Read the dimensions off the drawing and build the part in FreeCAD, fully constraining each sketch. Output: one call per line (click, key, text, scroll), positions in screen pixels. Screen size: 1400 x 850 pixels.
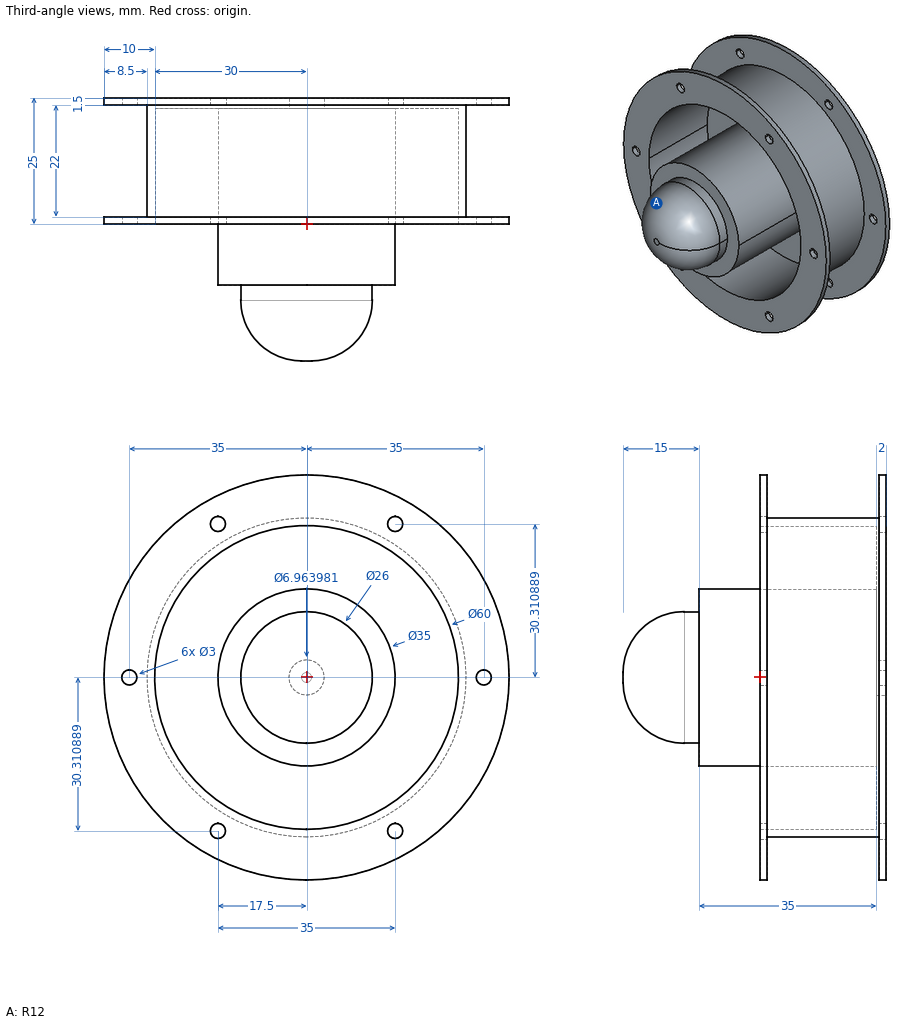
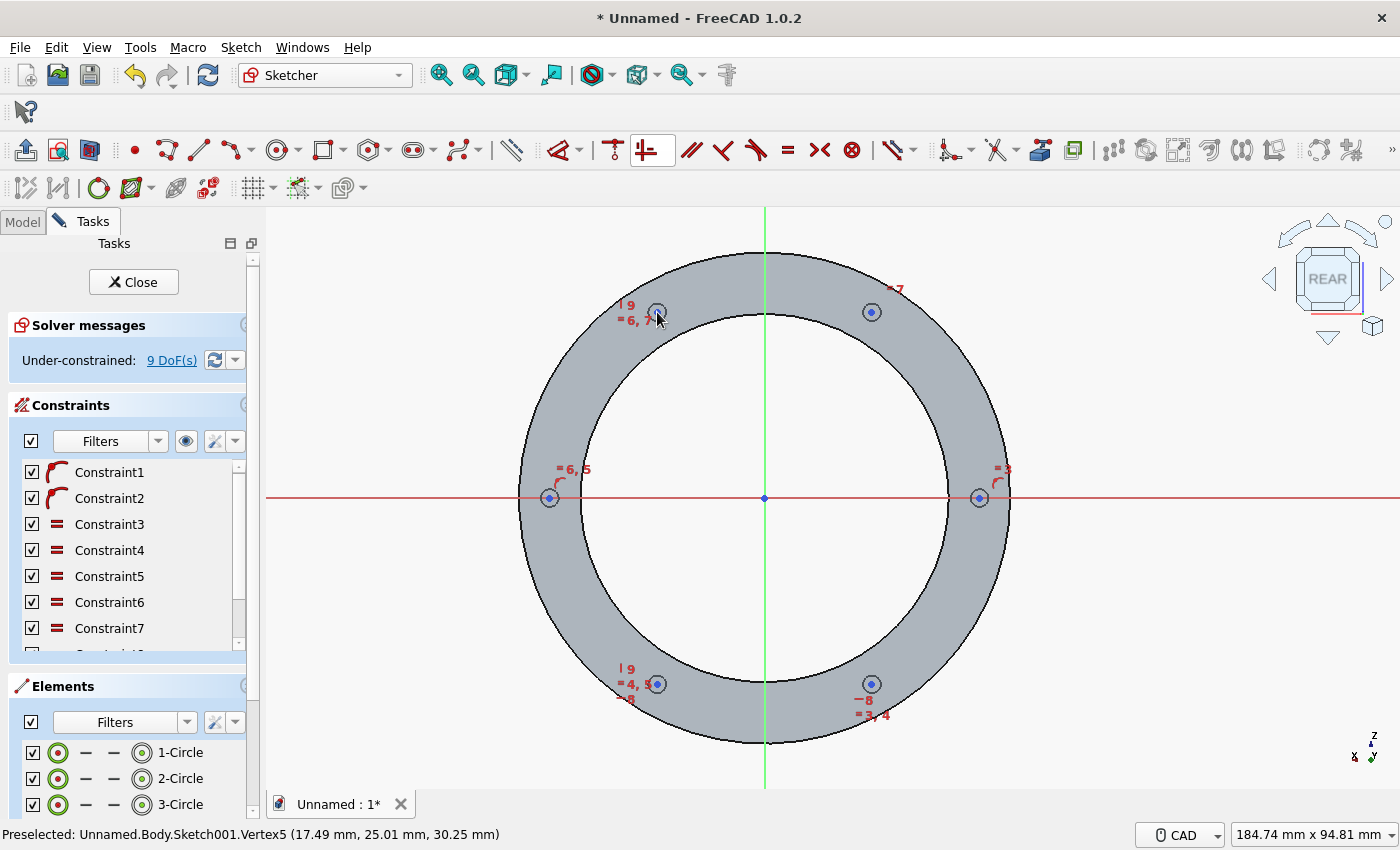
click(872, 684)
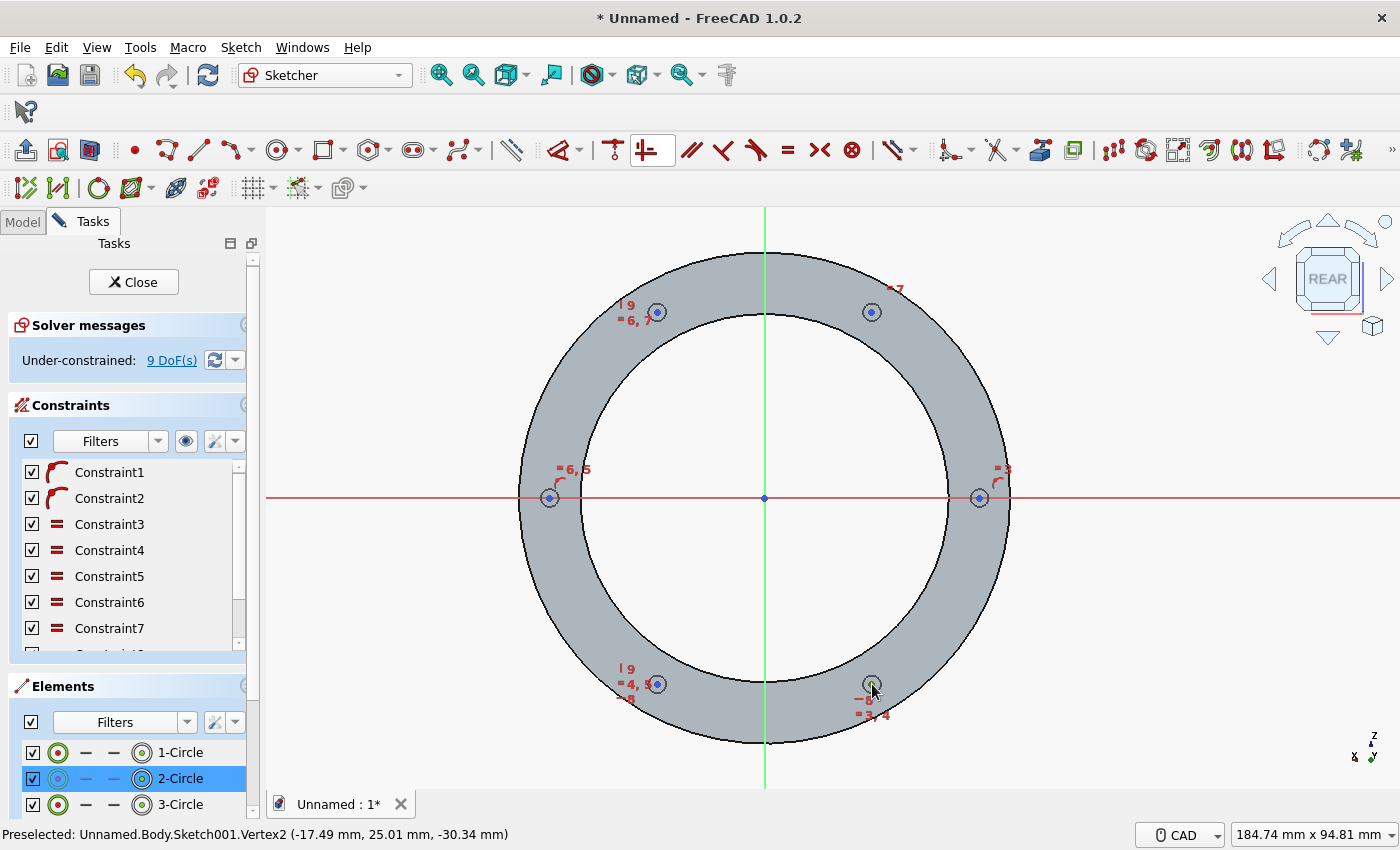
click(872, 312)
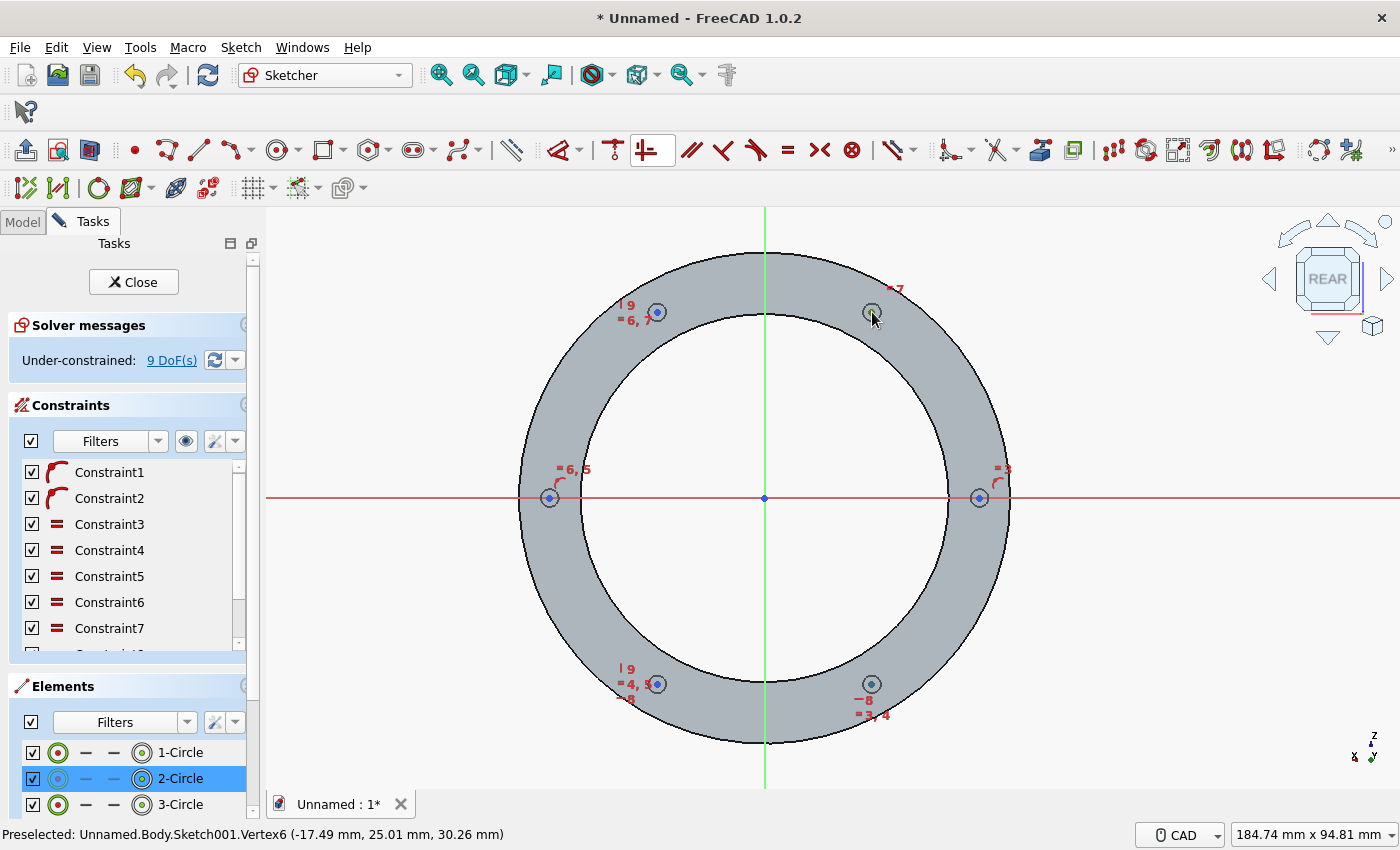
click(670, 150)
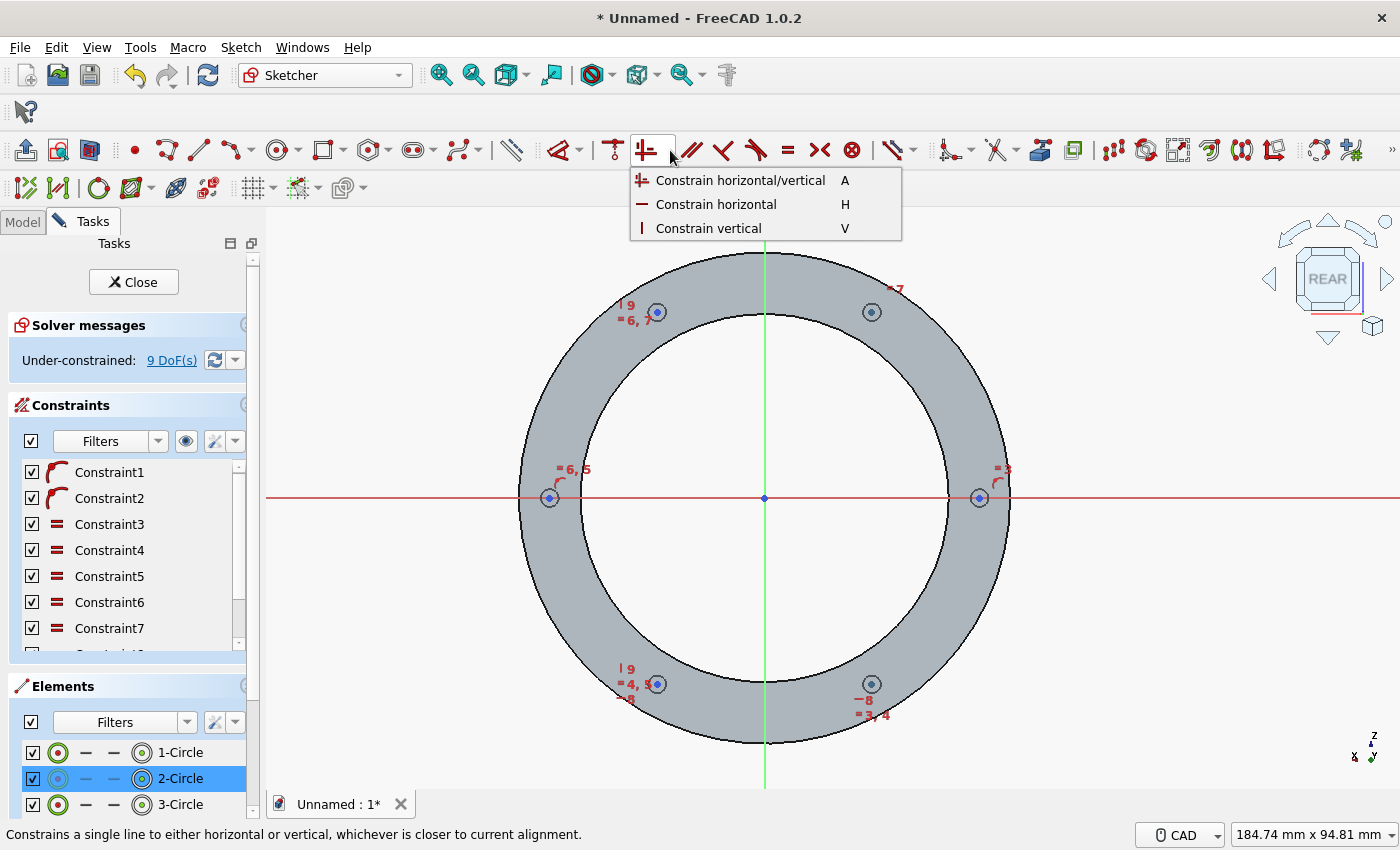
click(766, 228)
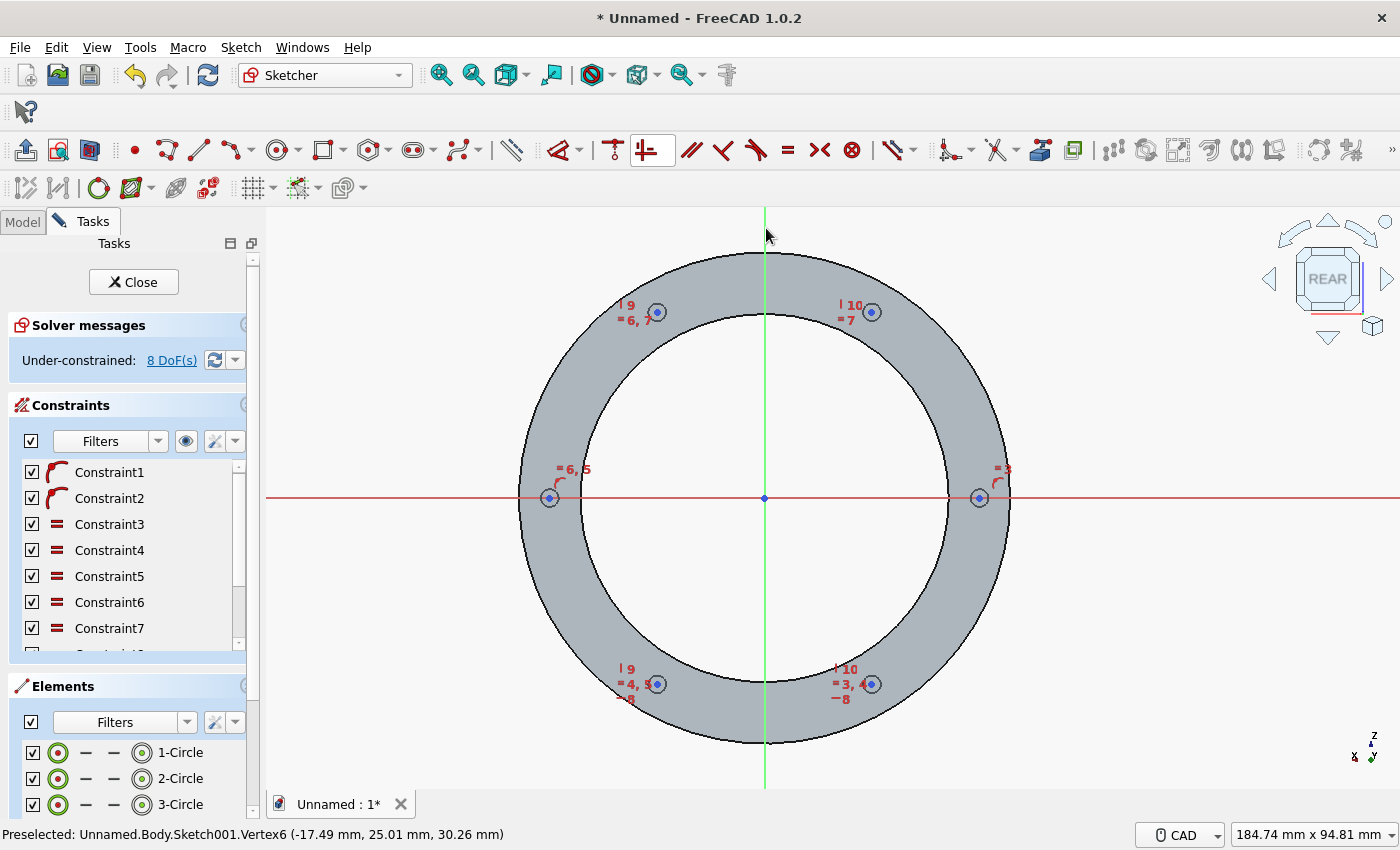
click(657, 312)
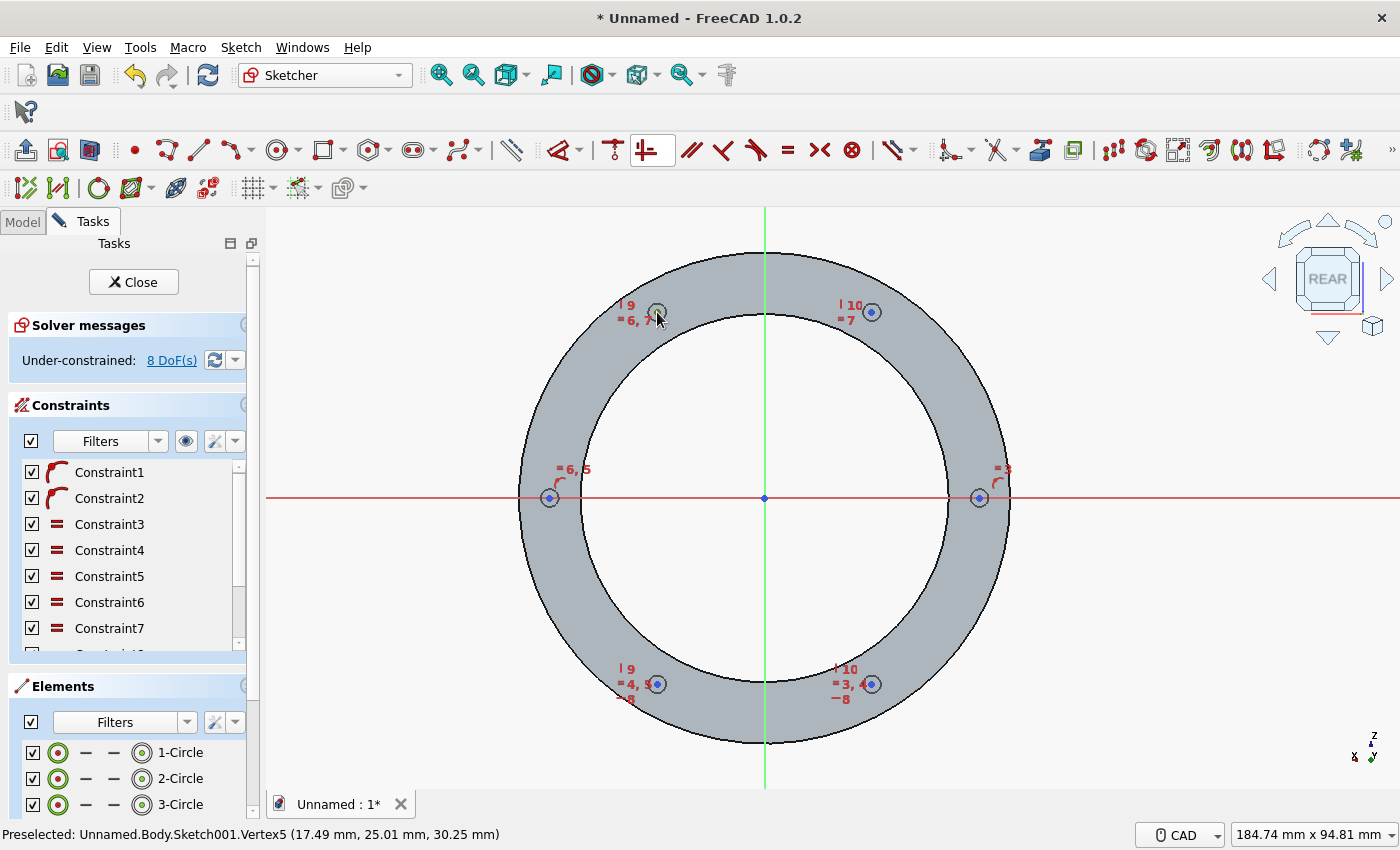
click(872, 312)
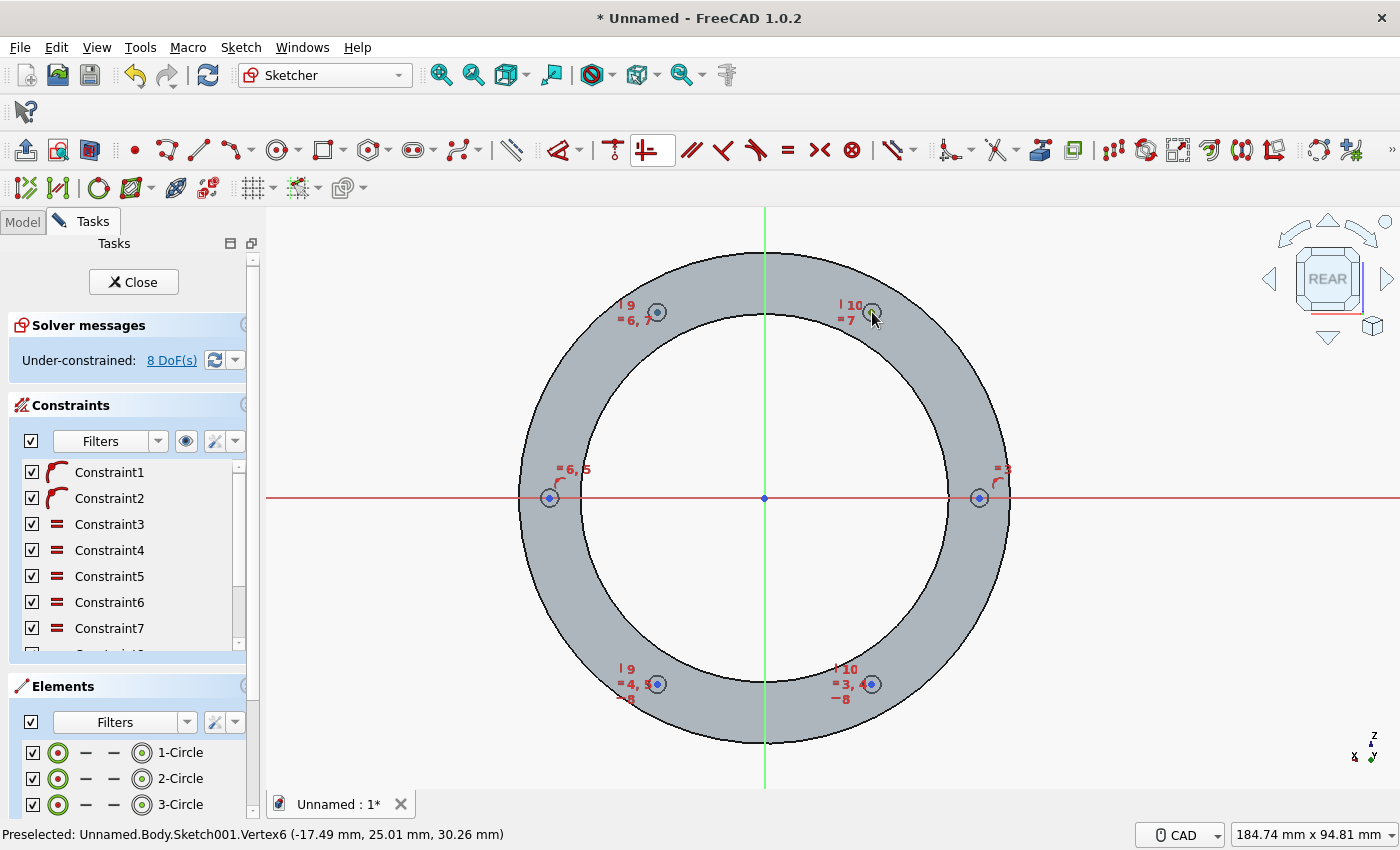
click(670, 150)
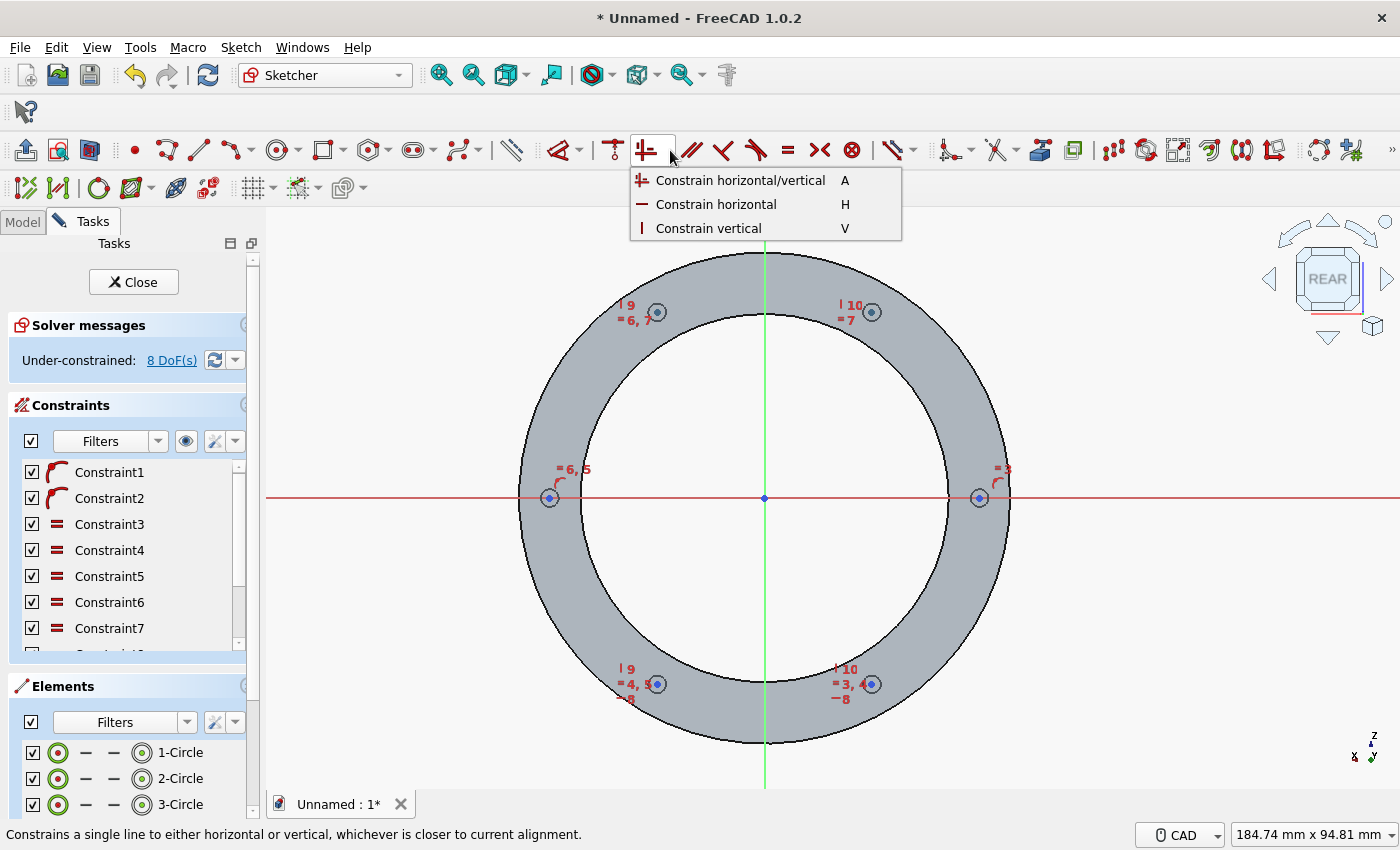
click(766, 204)